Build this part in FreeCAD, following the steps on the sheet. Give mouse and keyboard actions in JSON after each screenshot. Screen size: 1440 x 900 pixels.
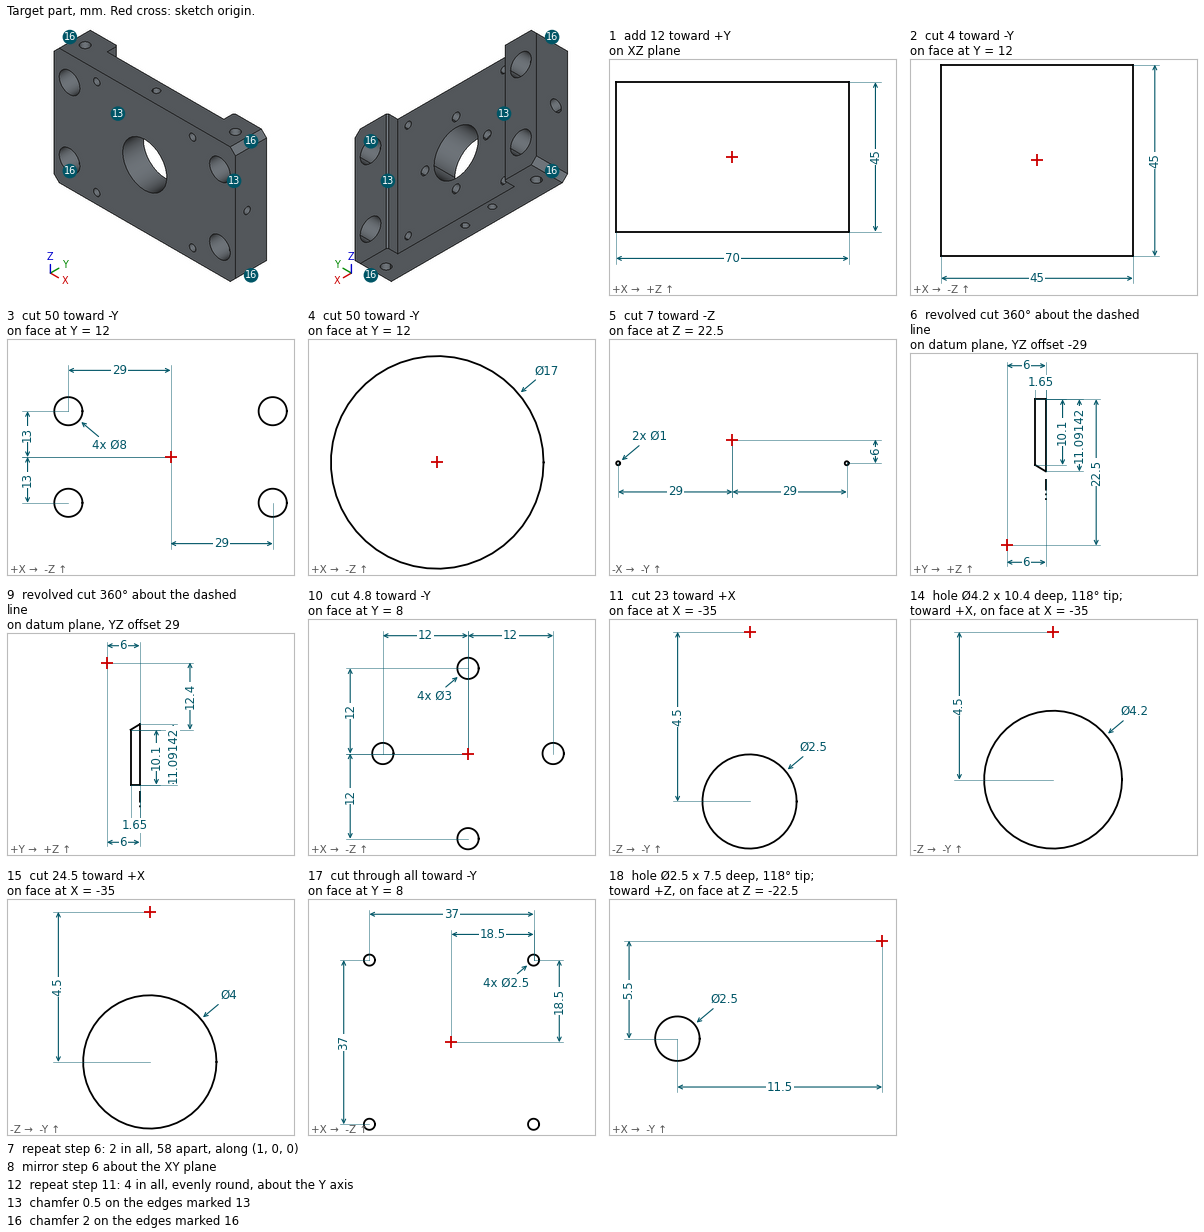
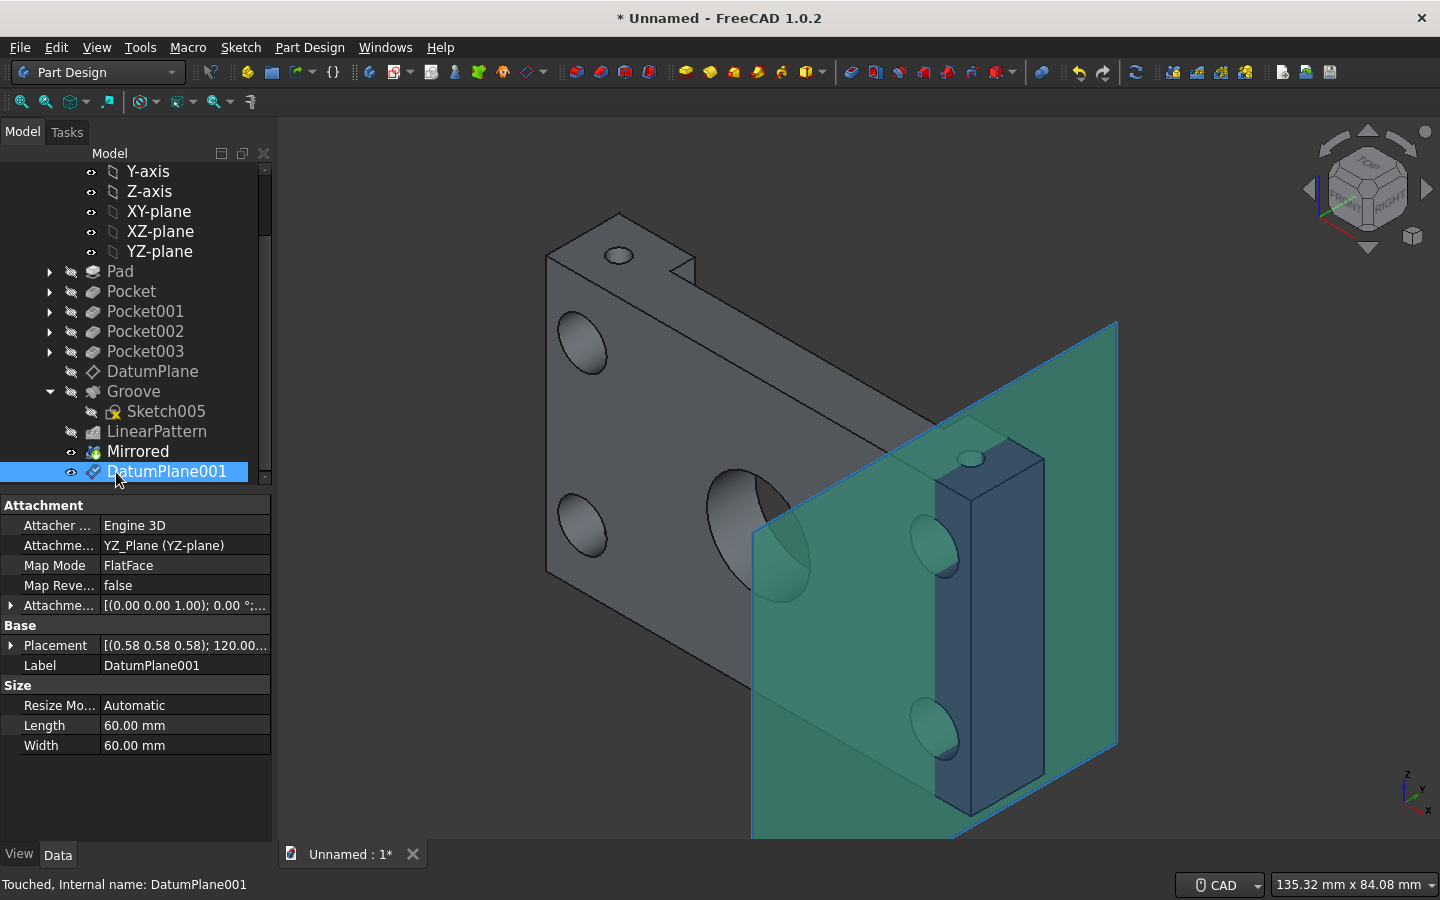
{"action": "left_click", "coordinate": [394, 72]}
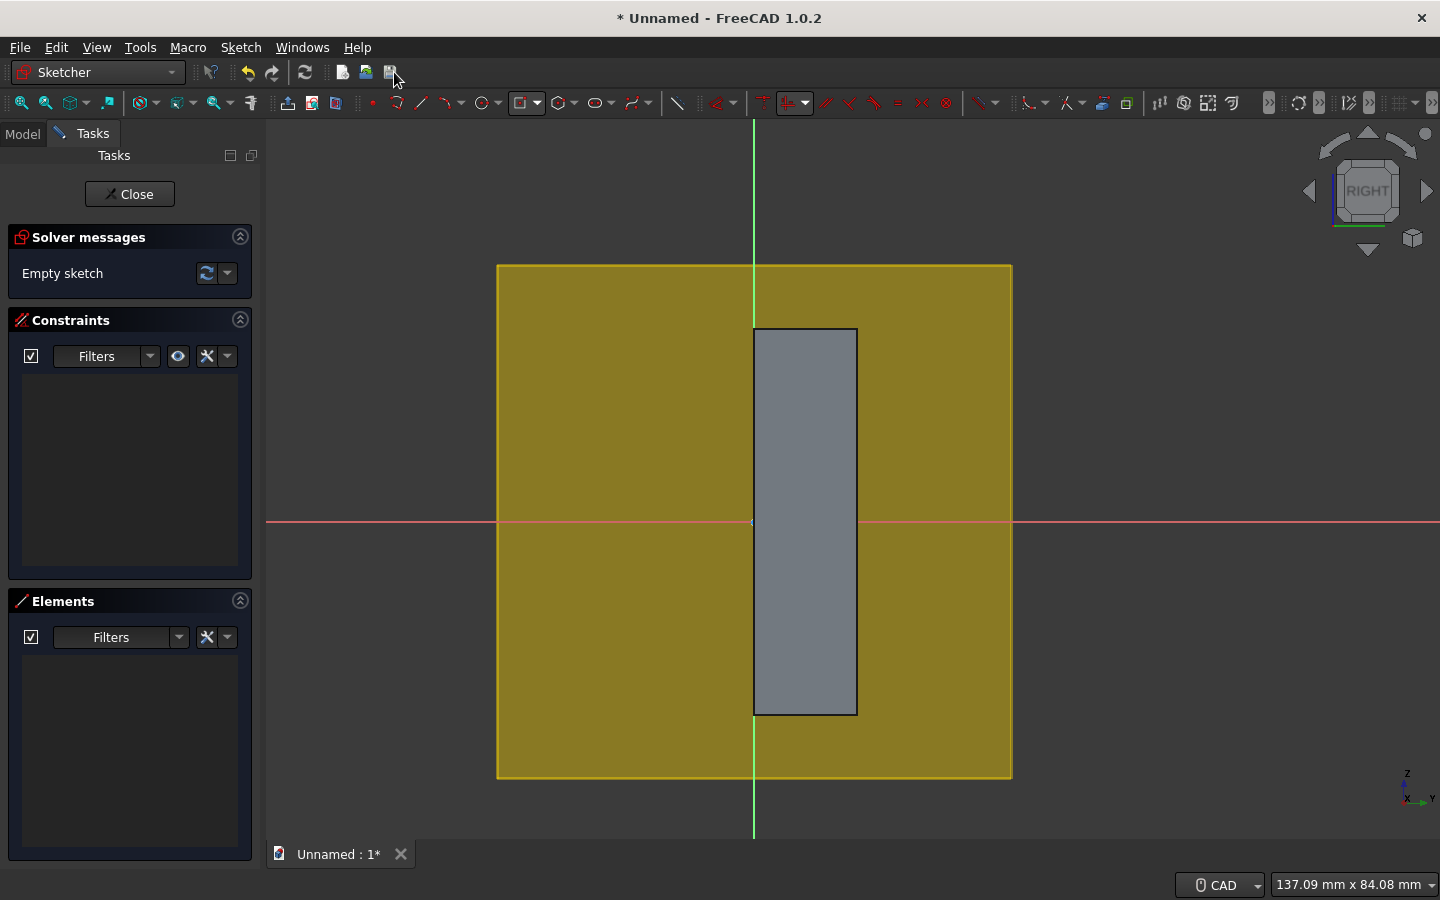
{"action": "left_click", "coordinate": [336, 104]}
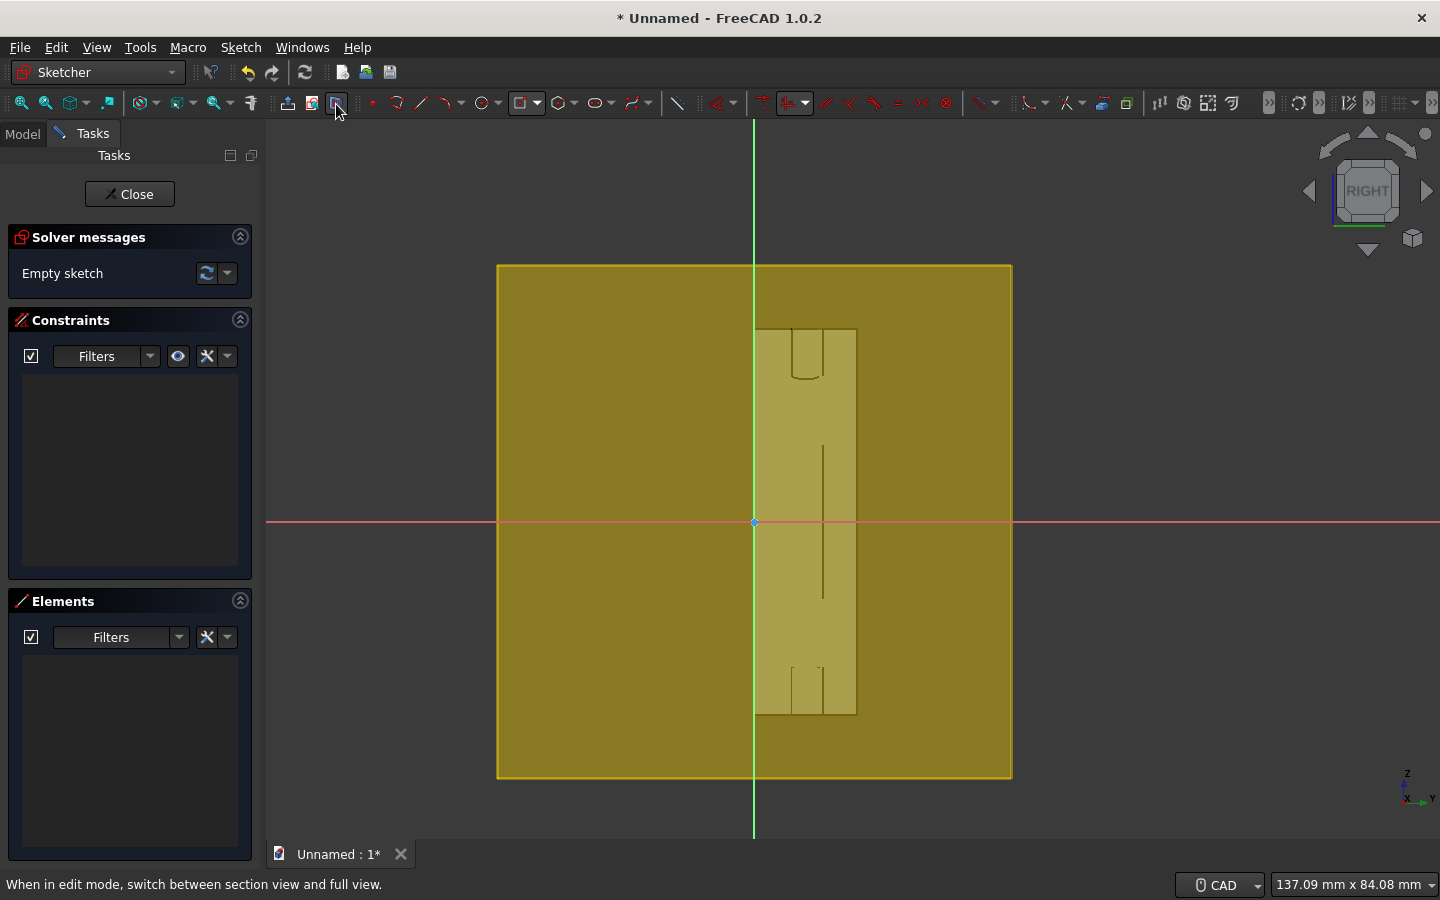
{"action": "scroll", "coordinate": [776, 767], "scroll_direction": "up", "scroll_amount": 4}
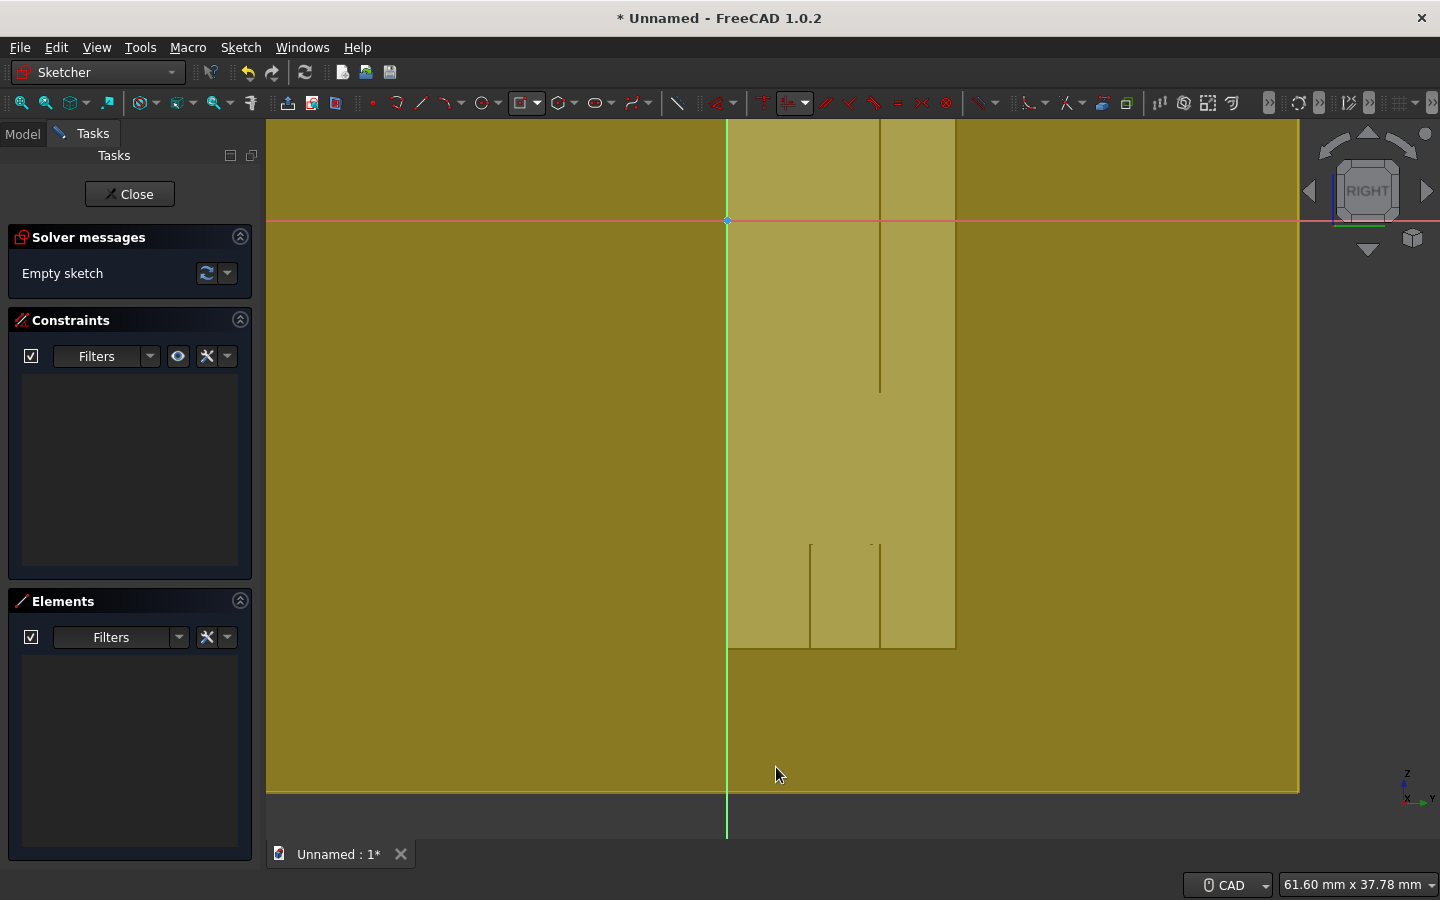
{"action": "left_click", "coordinate": [398, 104]}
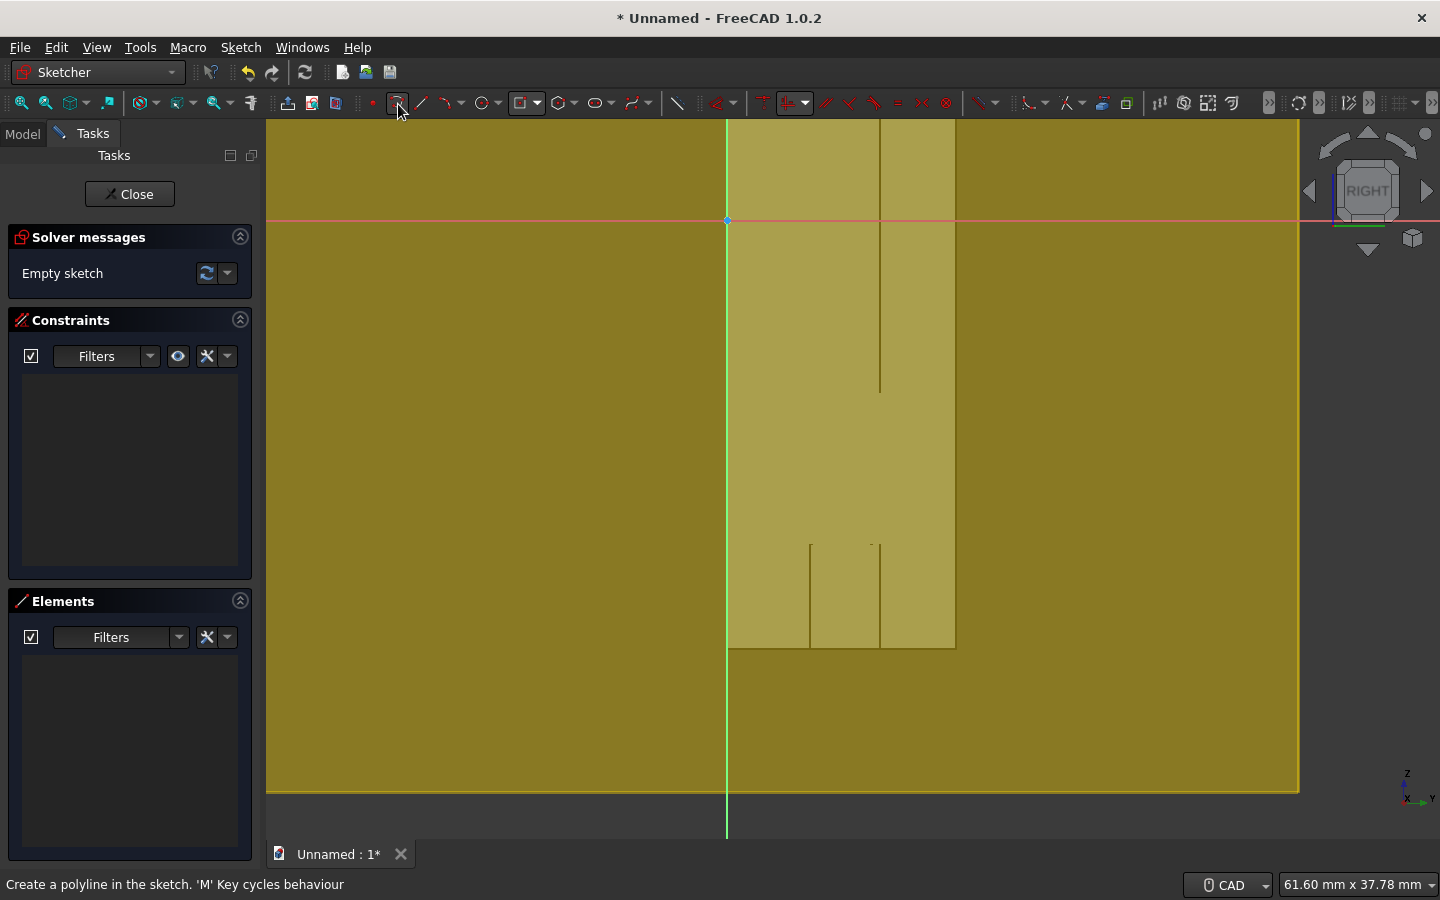
{"action": "left_click", "coordinate": [842, 438]}
{"action": "left_click", "coordinate": [810, 457]}
{"action": "left_click", "coordinate": [810, 649]}
{"action": "left_click", "coordinate": [842, 649]}
{"action": "left_click", "coordinate": [842, 439]}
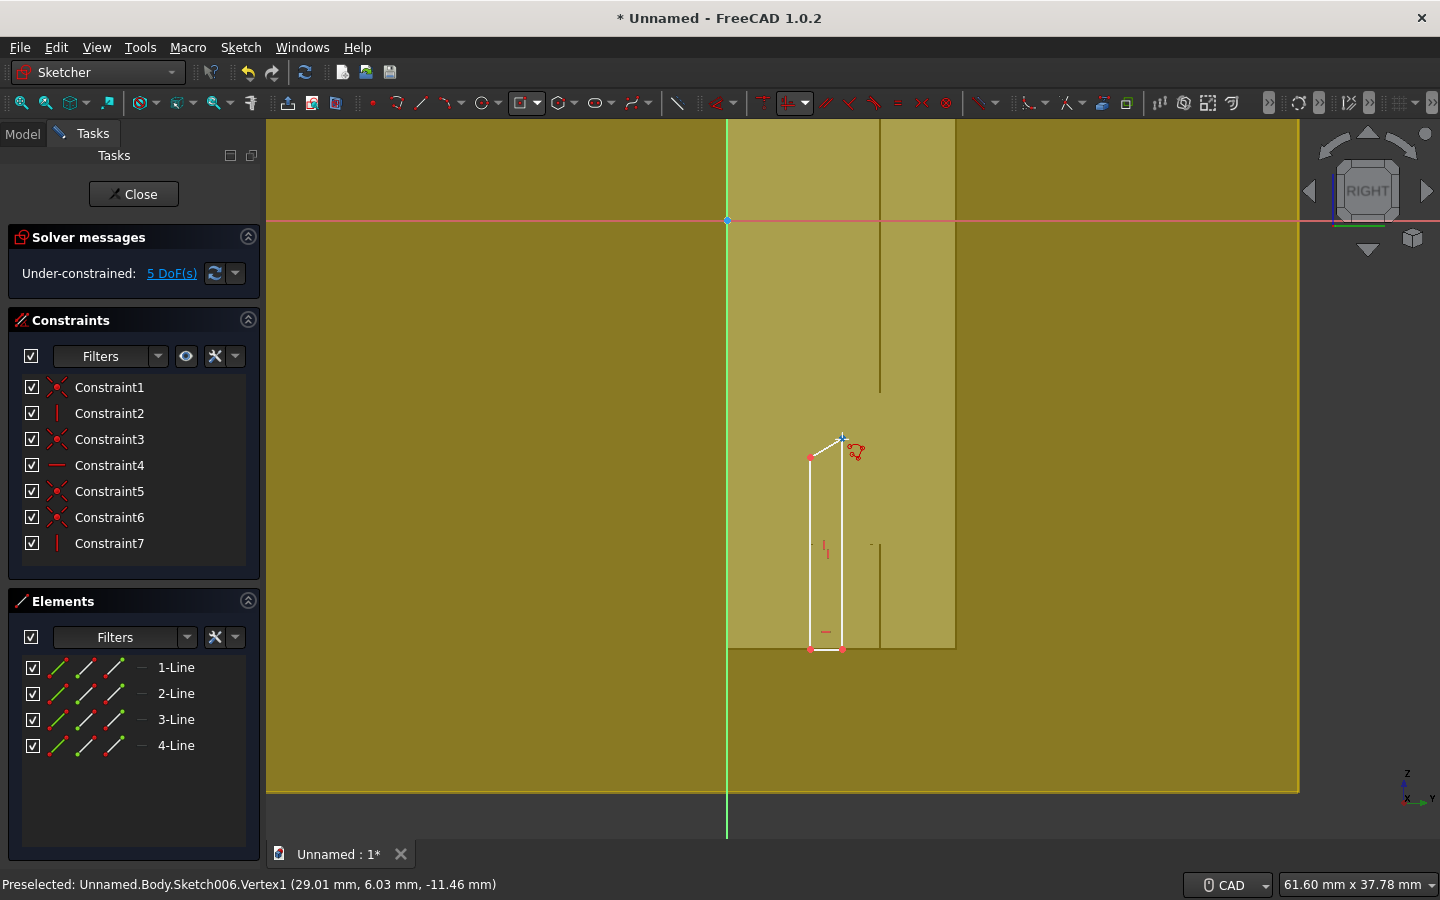
{"action": "left_click", "coordinate": [422, 104]}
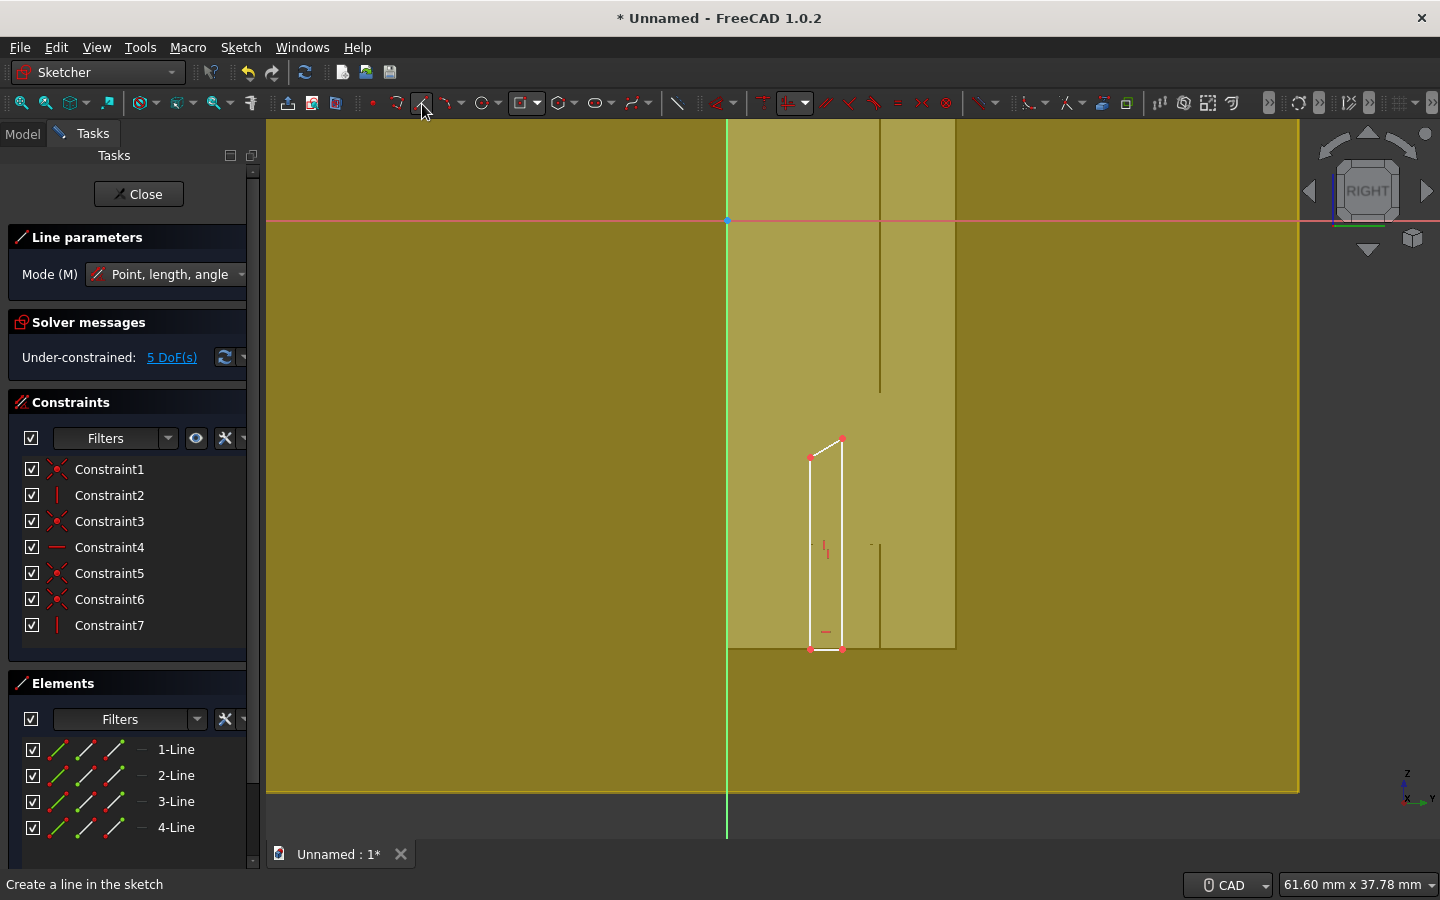
{"action": "left_click", "coordinate": [842, 671]}
{"action": "left_click", "coordinate": [842, 734]}
{"action": "key", "text": "Escape"}